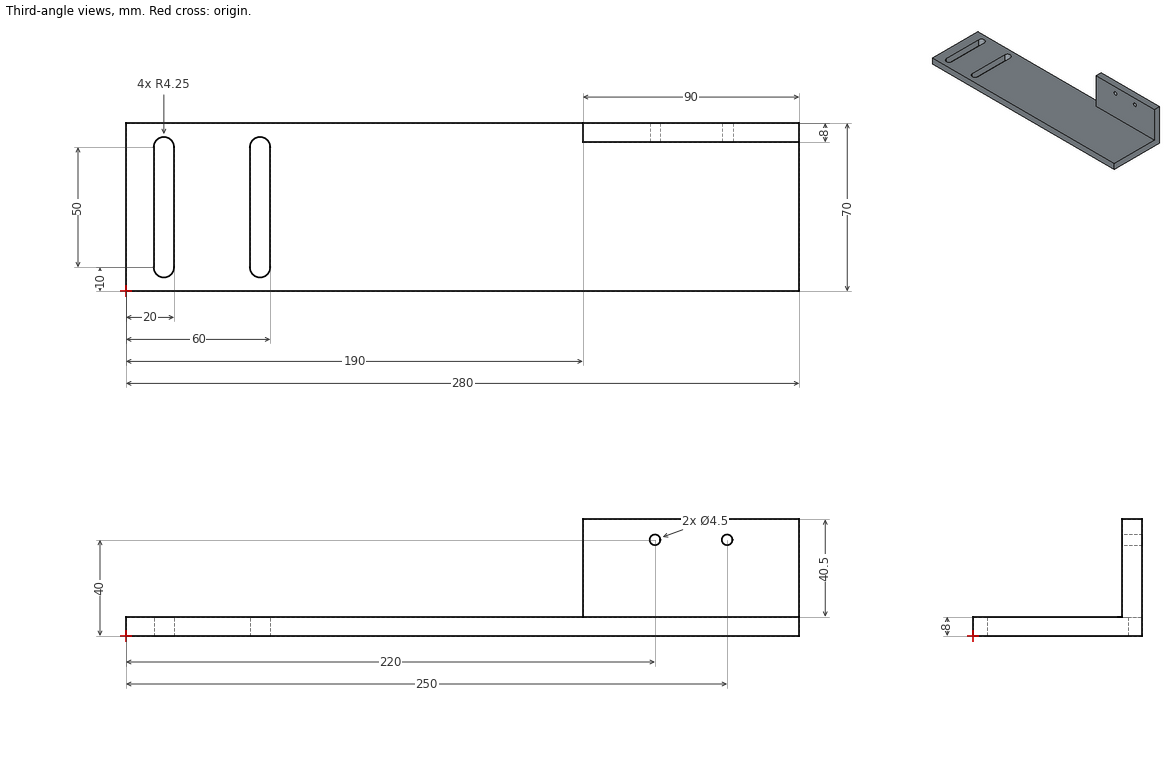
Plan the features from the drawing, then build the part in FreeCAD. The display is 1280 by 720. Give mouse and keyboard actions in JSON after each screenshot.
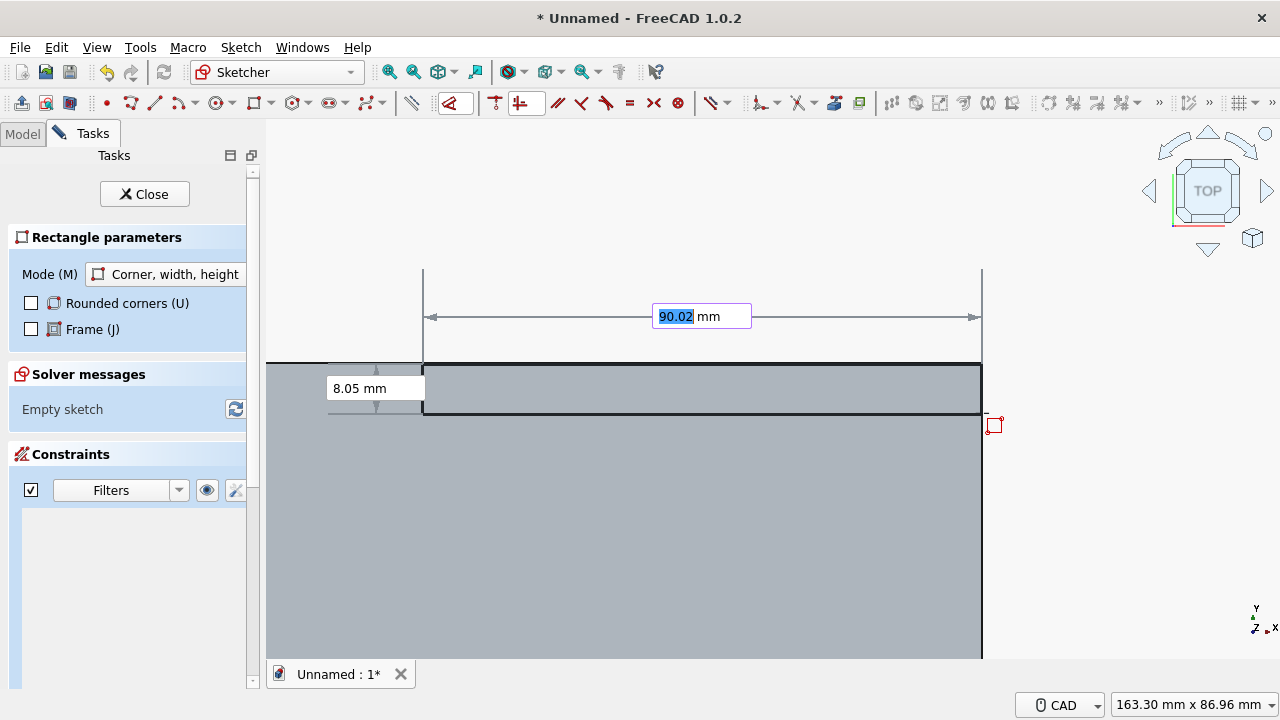
{"action": "type", "text": "90"}
{"action": "key", "text": "Tab"}
{"action": "type", "text": "8"}
{"action": "key", "text": "Return"}
{"action": "key", "text": "Escape"}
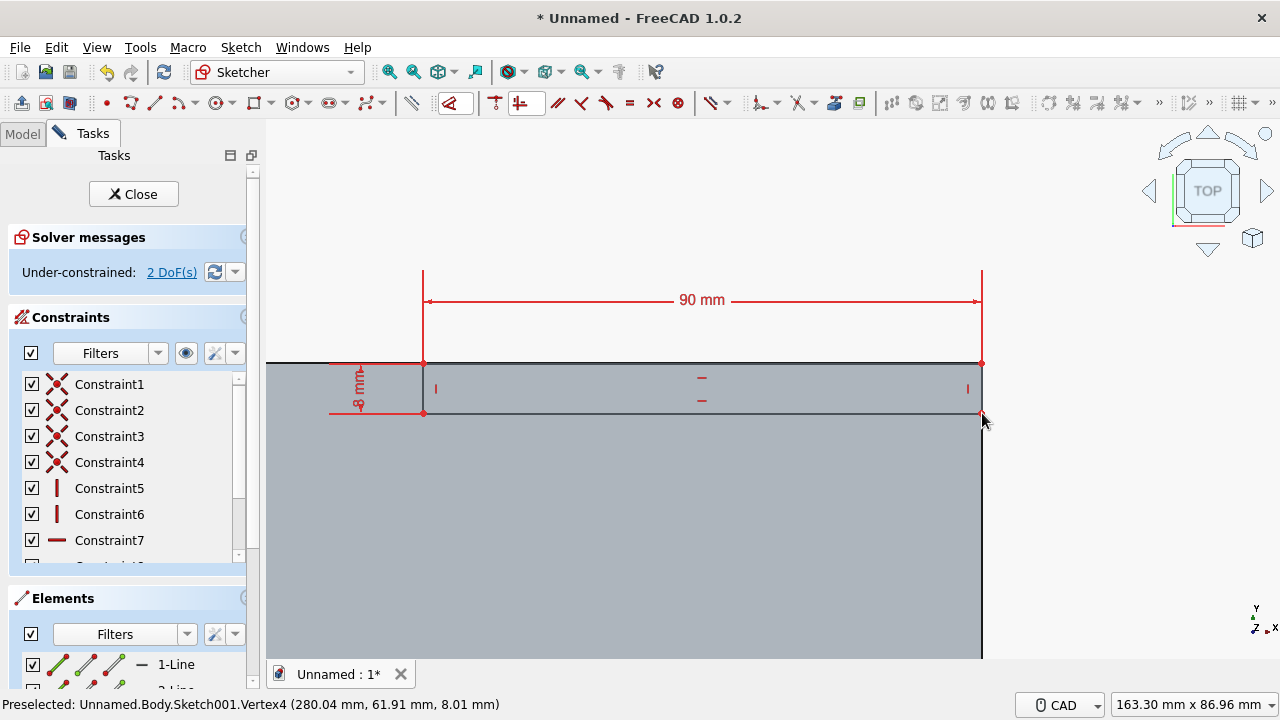
{"action": "left_click", "coordinate": [423, 364]}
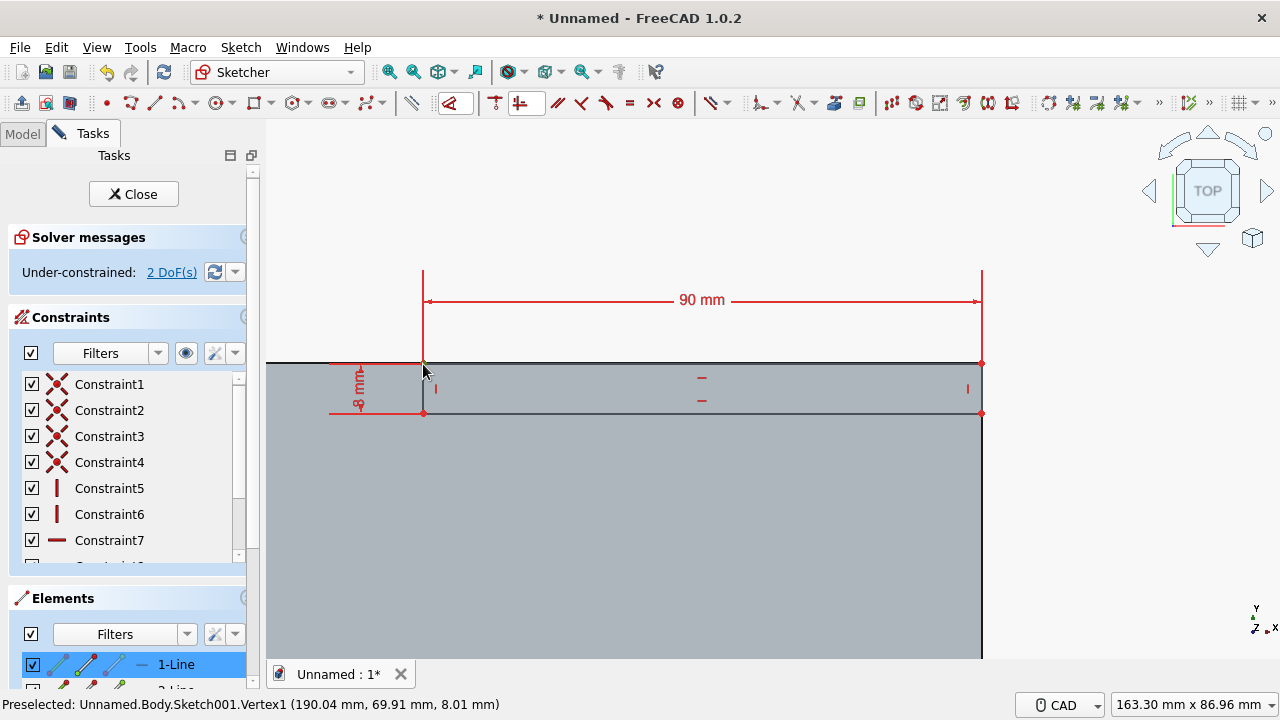
{"action": "key", "text": "i"}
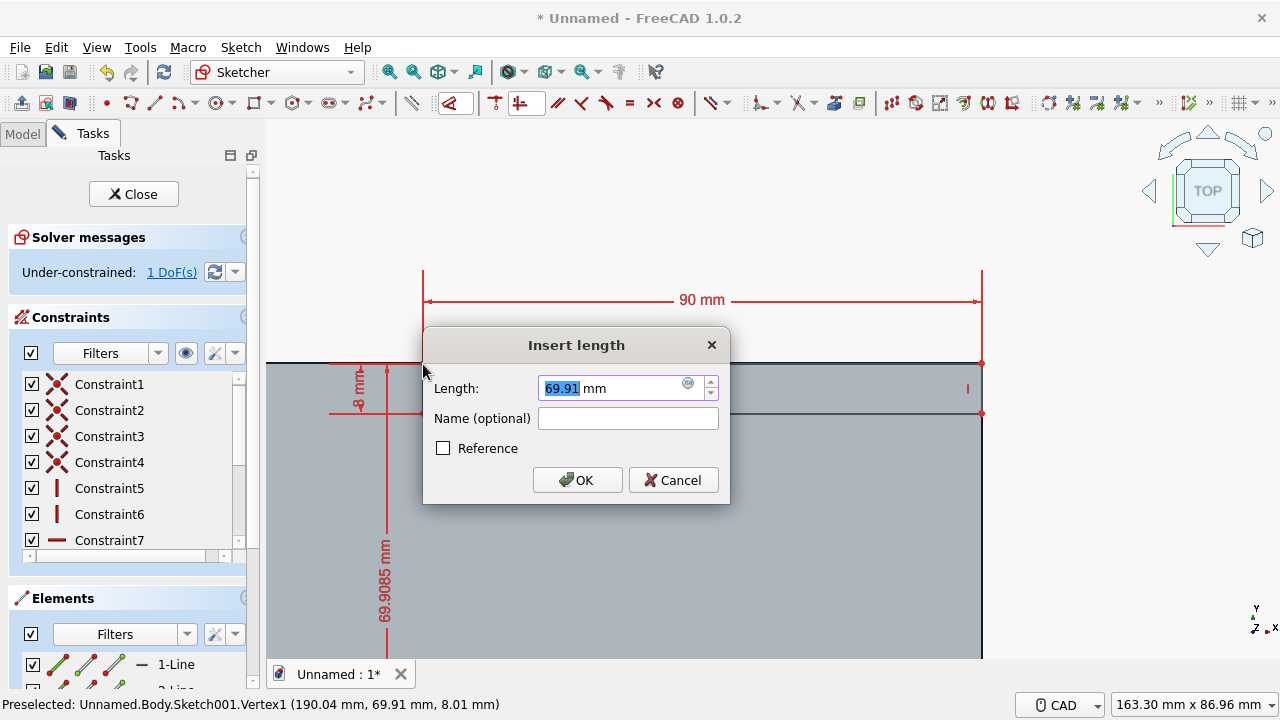
{"action": "type", "text": "70"}
{"action": "key", "text": "Return"}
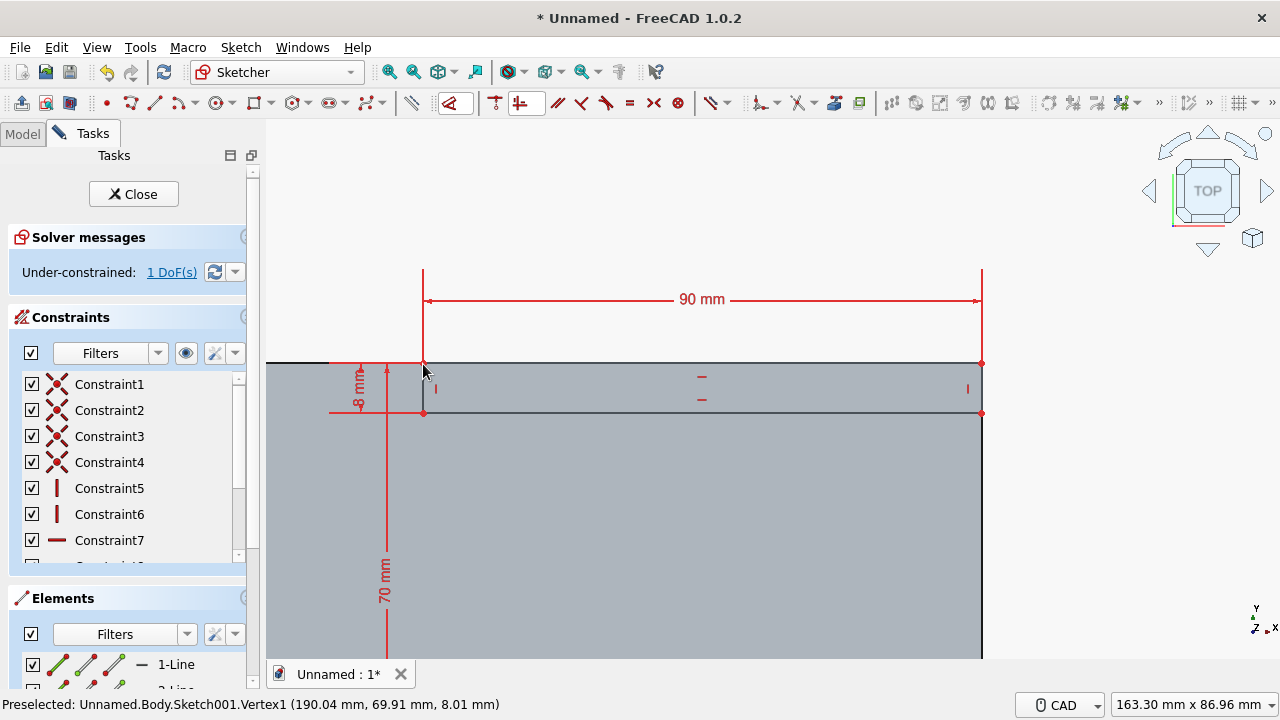
{"action": "left_click", "coordinate": [423, 363]}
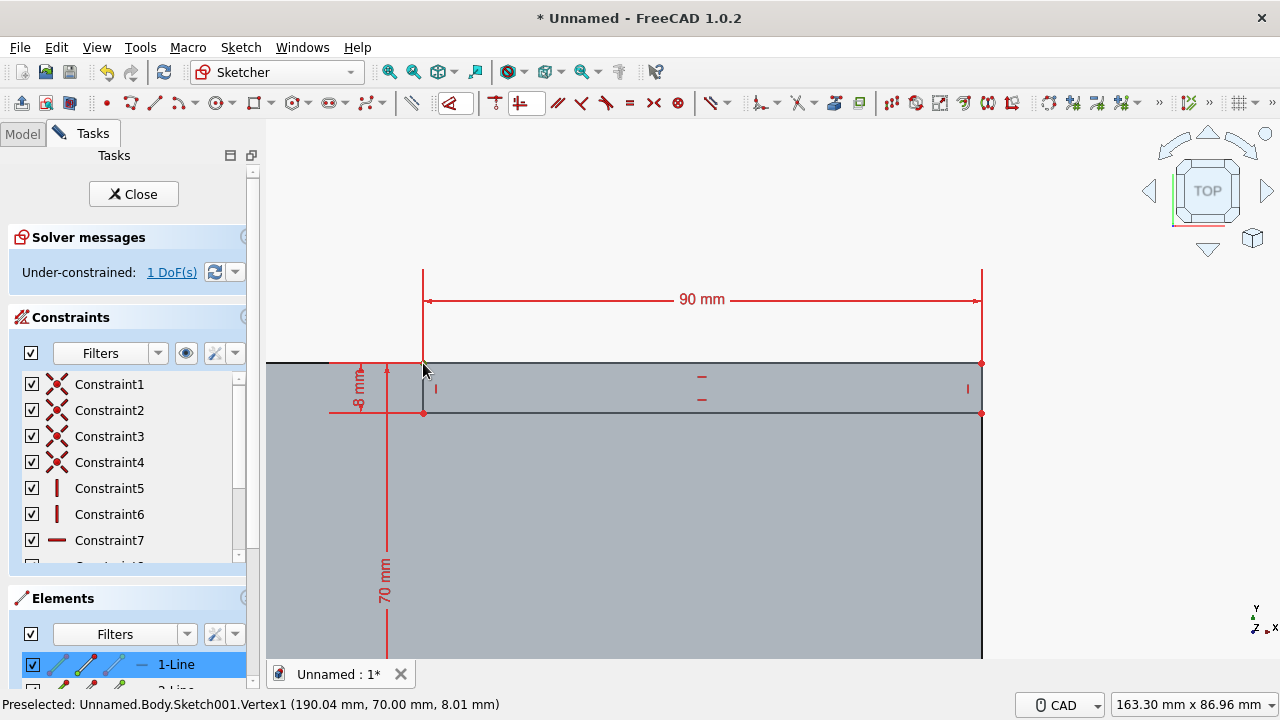
{"action": "key", "text": "l"}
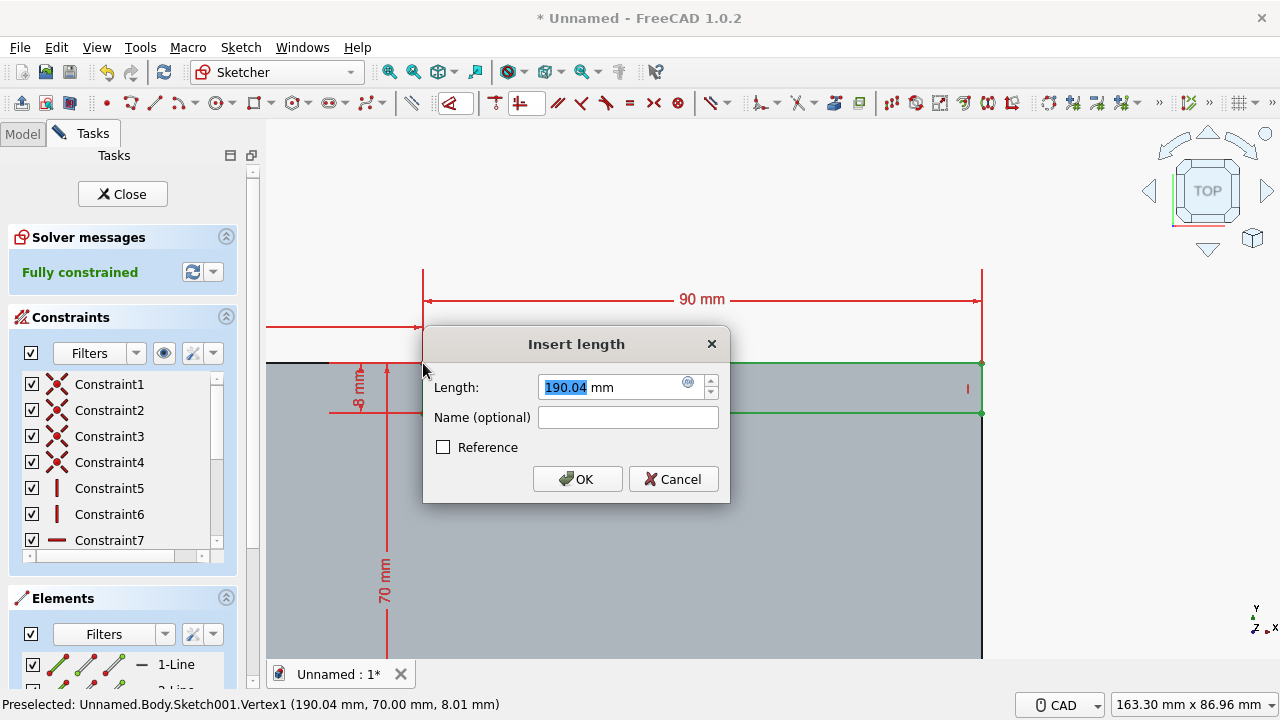
{"action": "type", "text": "190"}
{"action": "key", "text": "Return"}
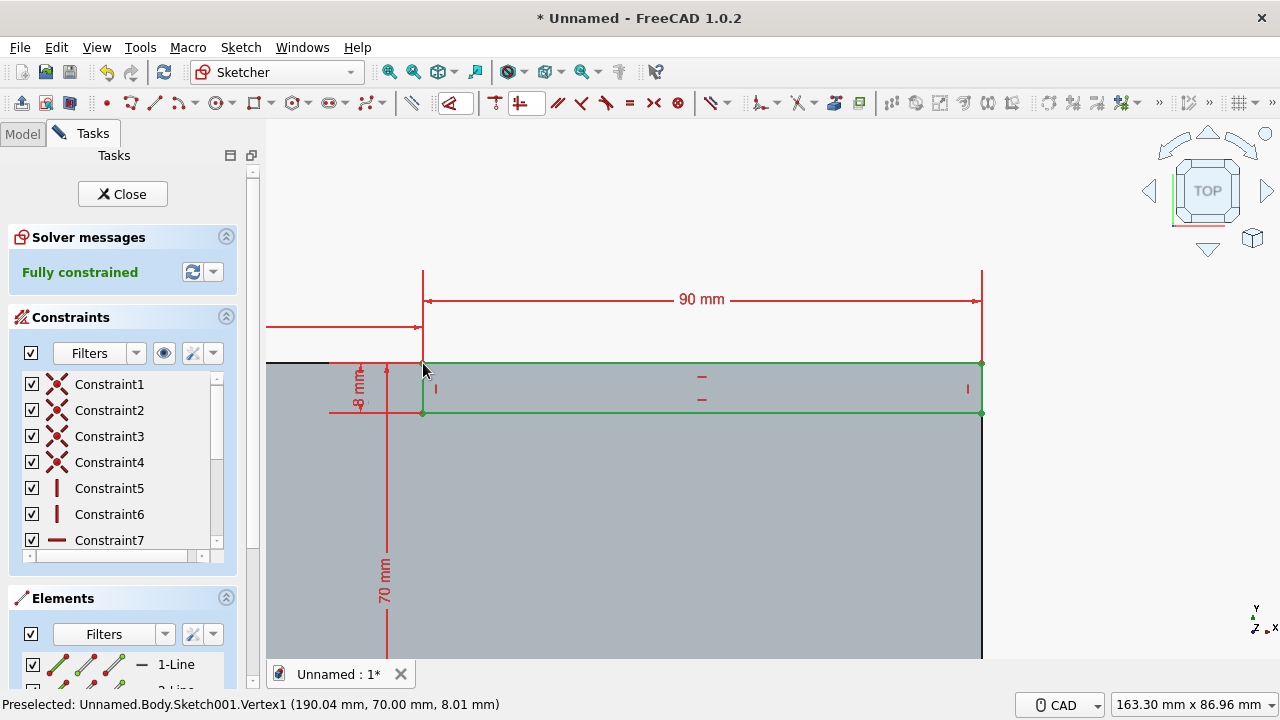
{"action": "left_click", "coordinate": [123, 194]}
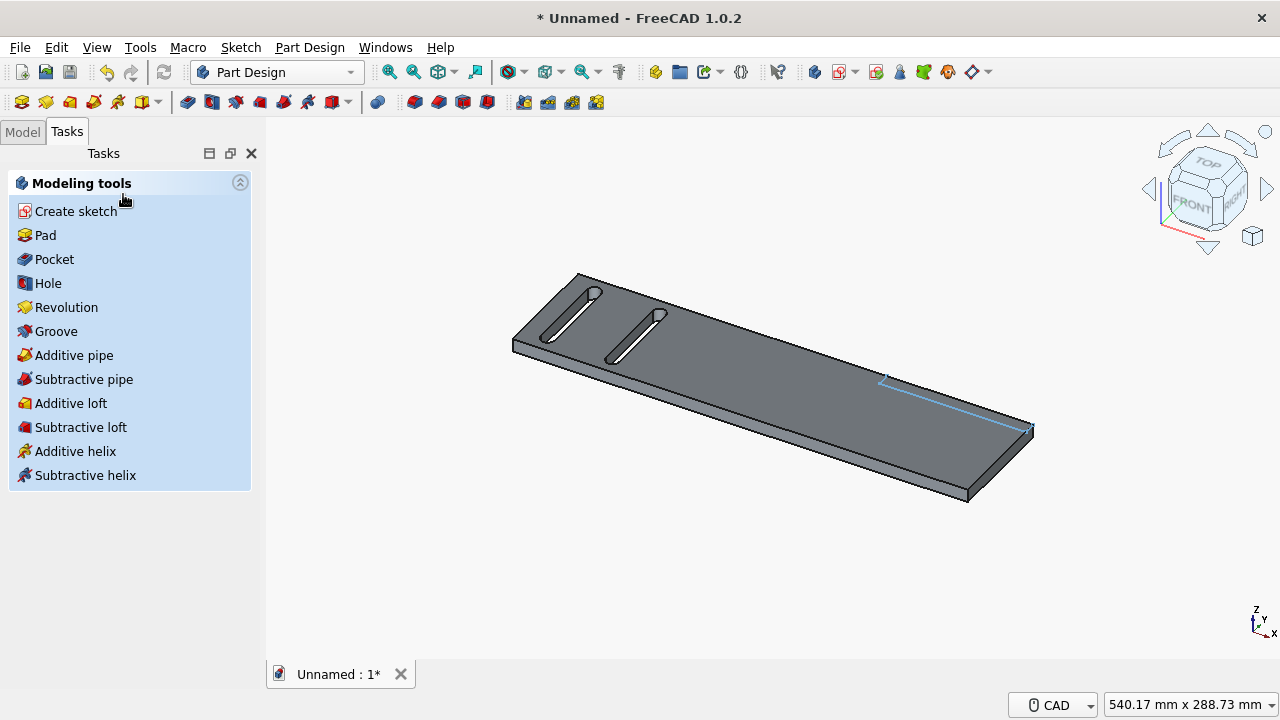
{"action": "left_click", "coordinate": [22, 102]}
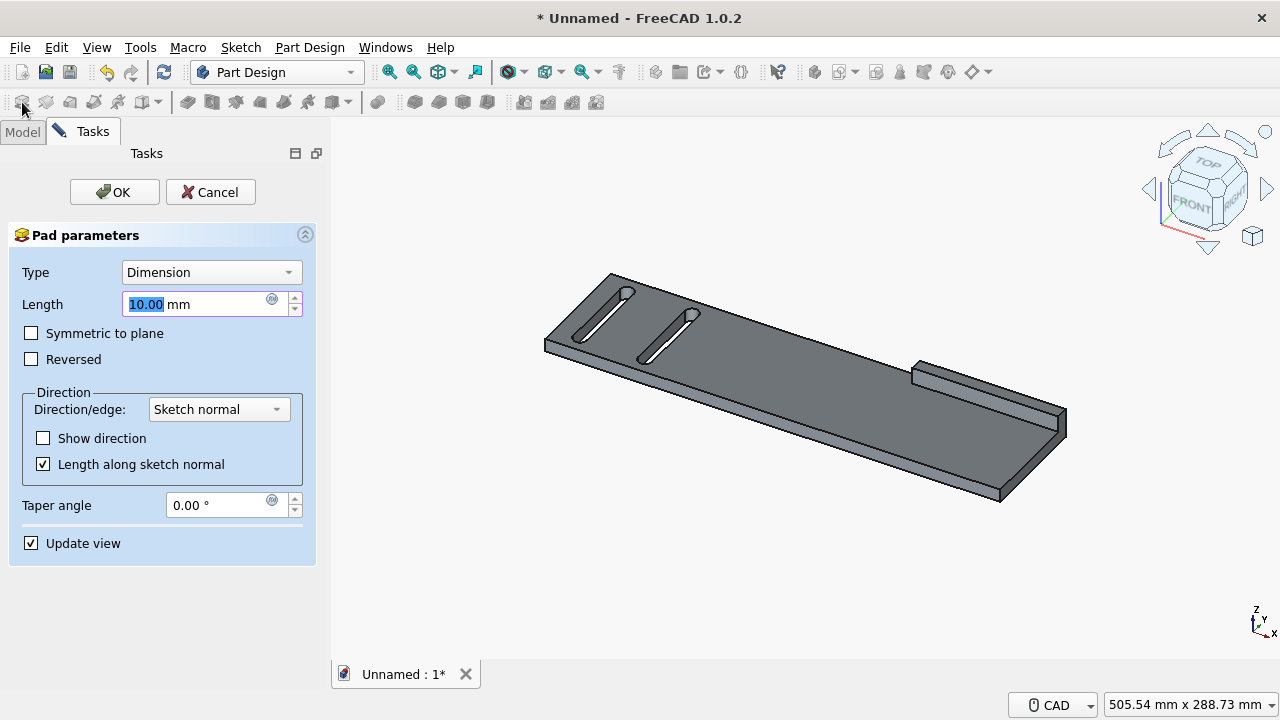
{"action": "type", "text": "40.5"}
{"action": "key", "text": "Tab"}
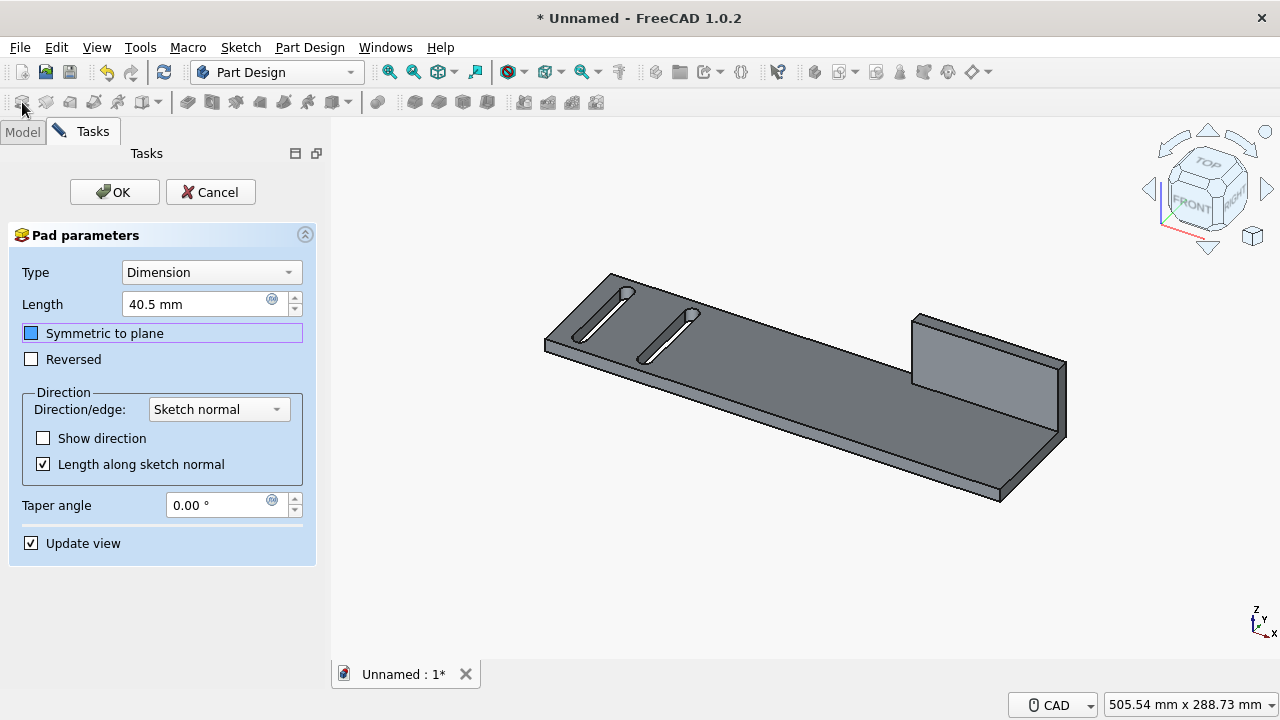
{"action": "left_click", "coordinate": [115, 192]}